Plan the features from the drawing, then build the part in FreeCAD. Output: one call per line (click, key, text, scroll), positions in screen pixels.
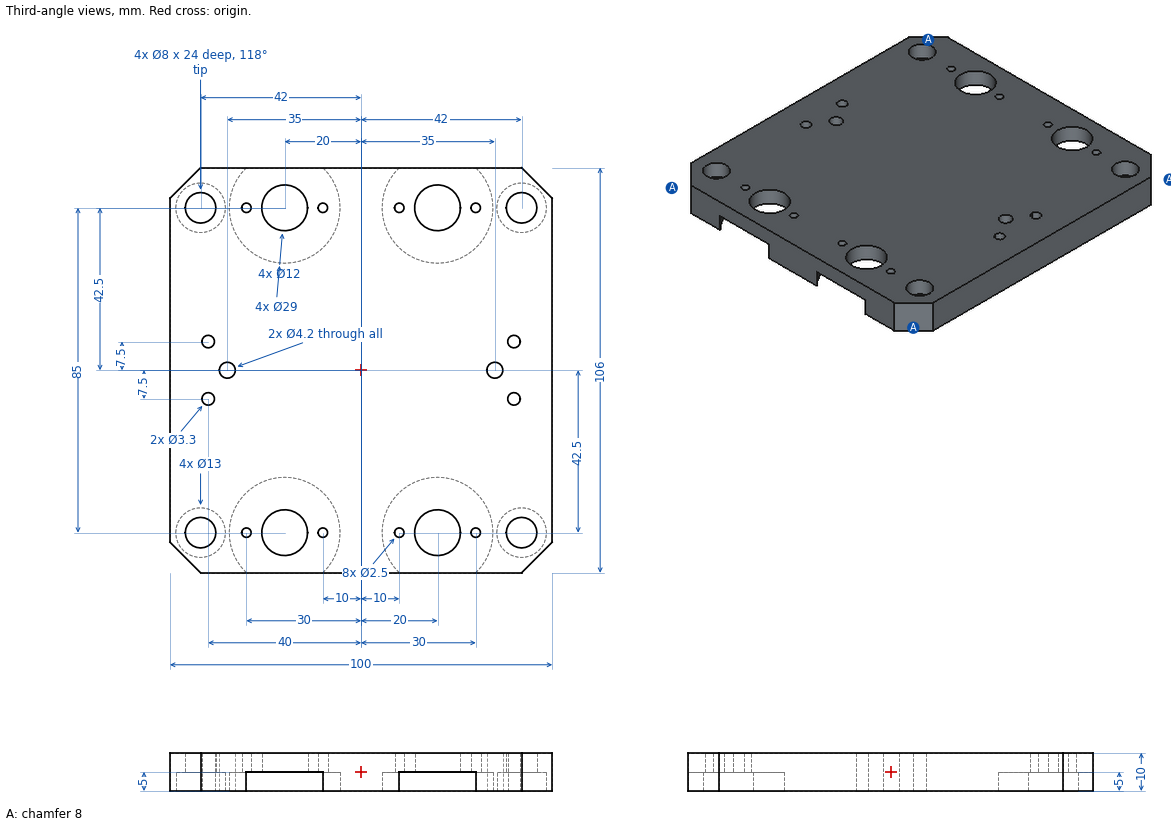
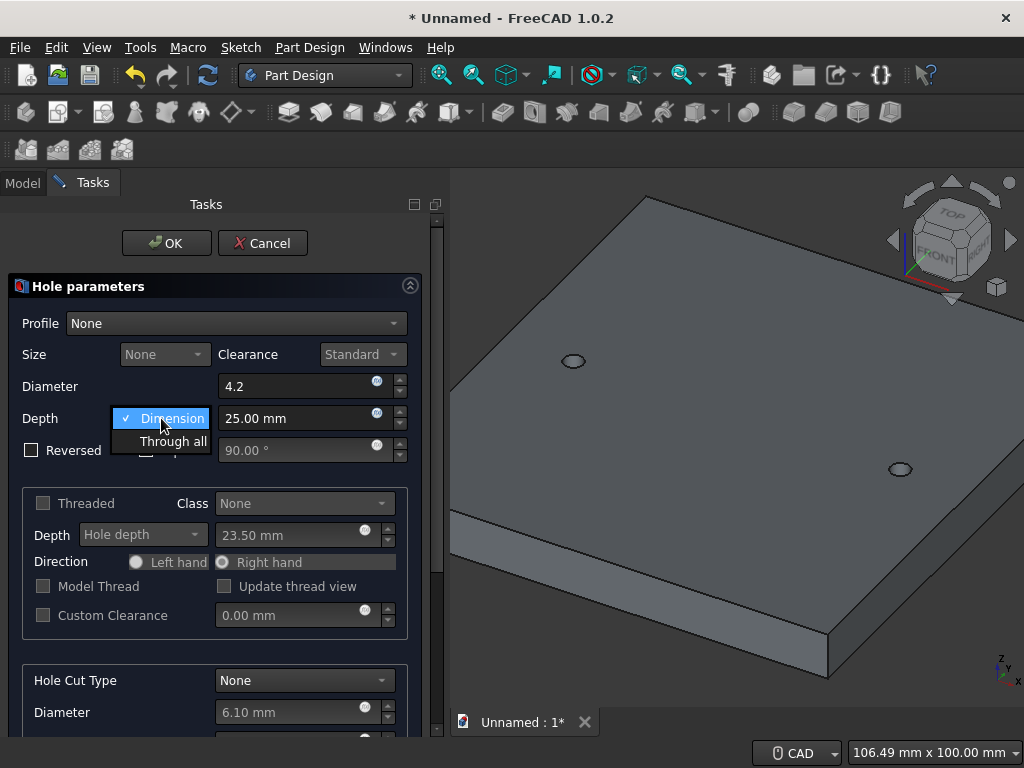
click(160, 442)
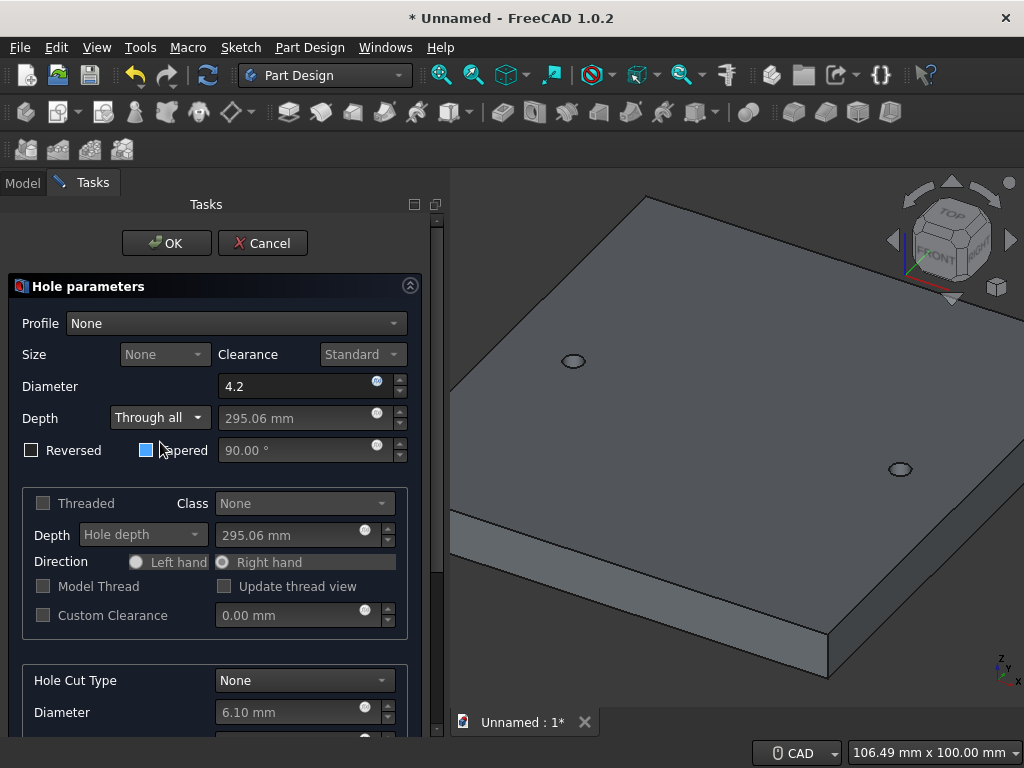
click(167, 243)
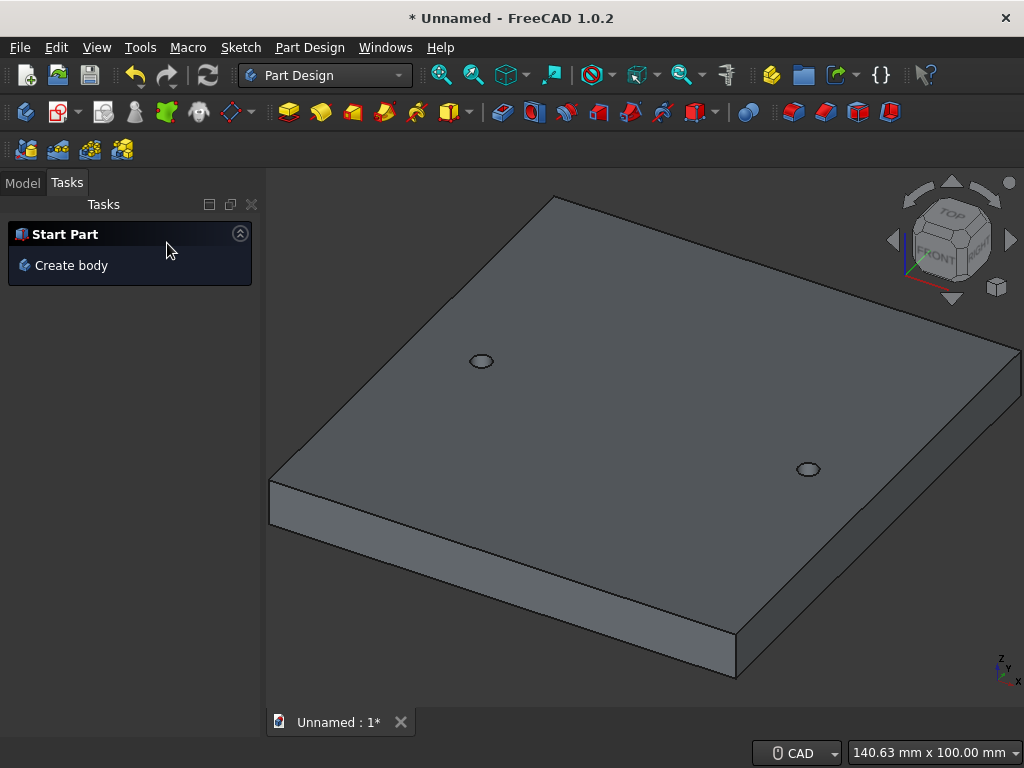
click(736, 656)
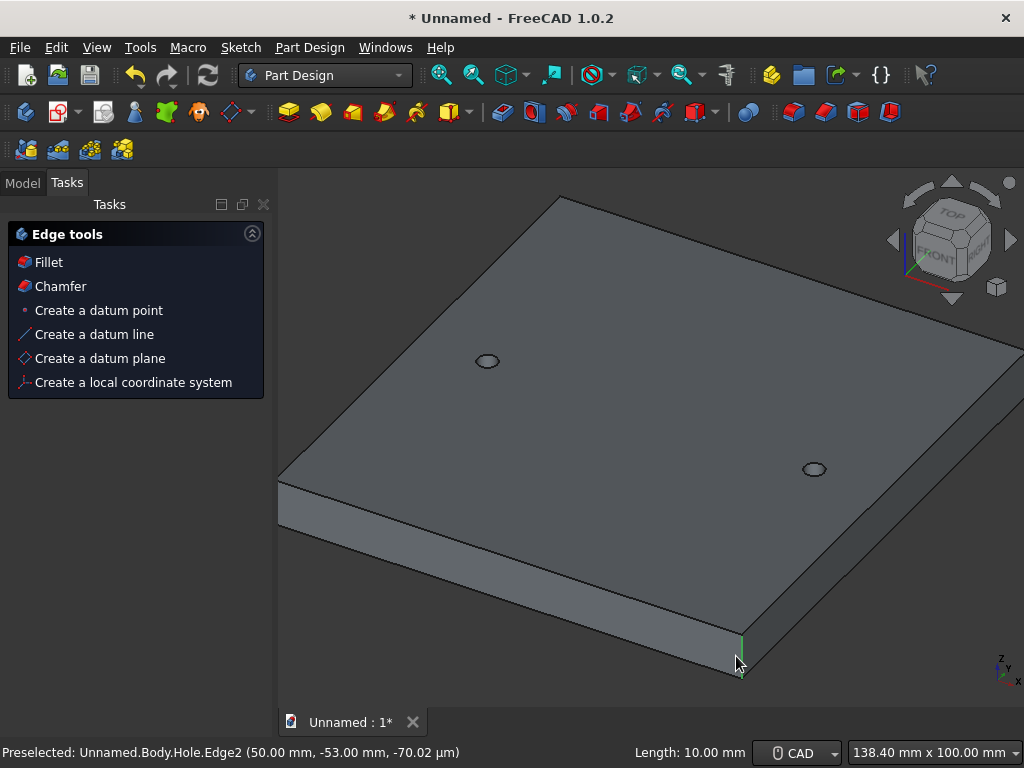
key(0)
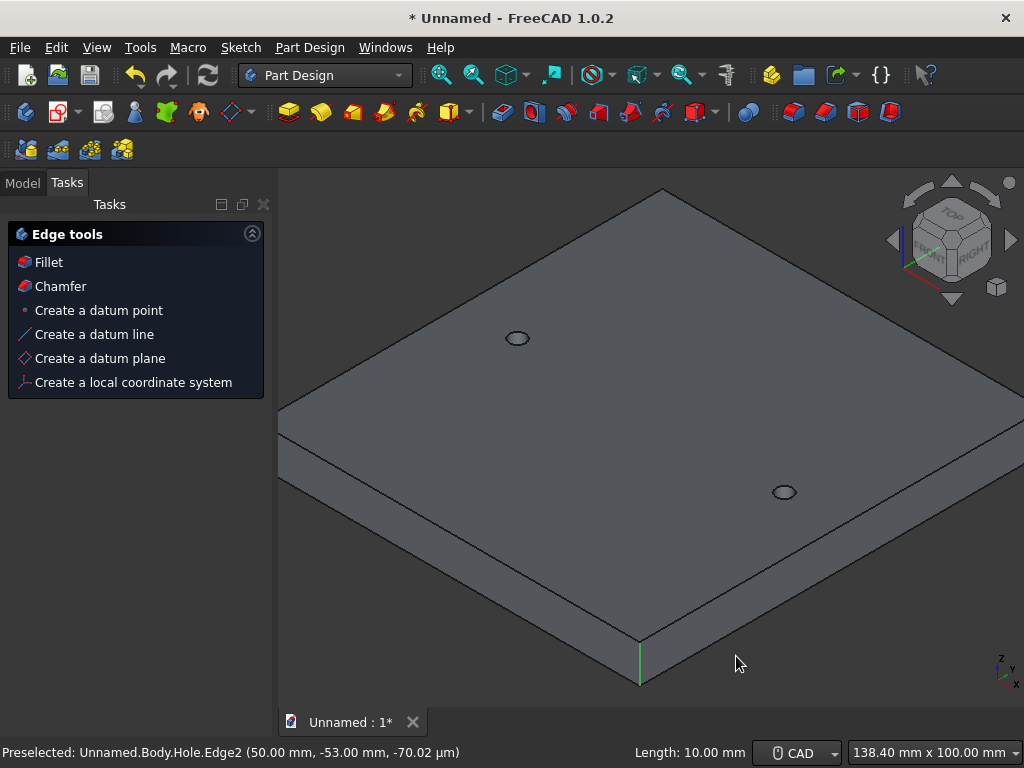
click(442, 76)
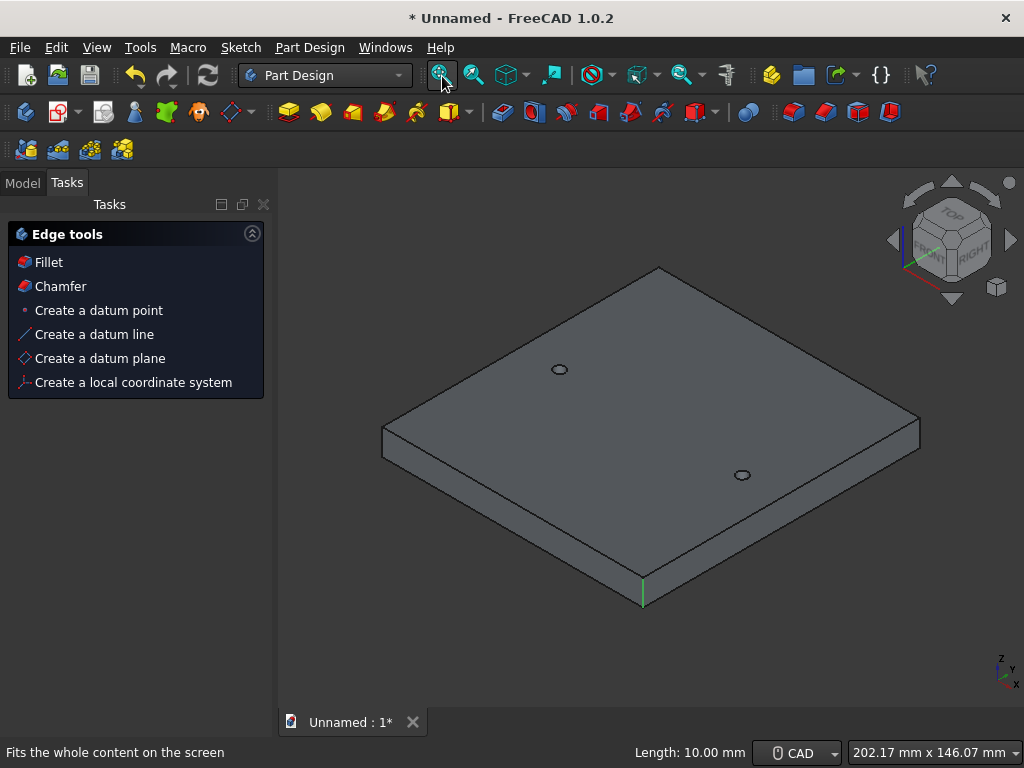
key(2)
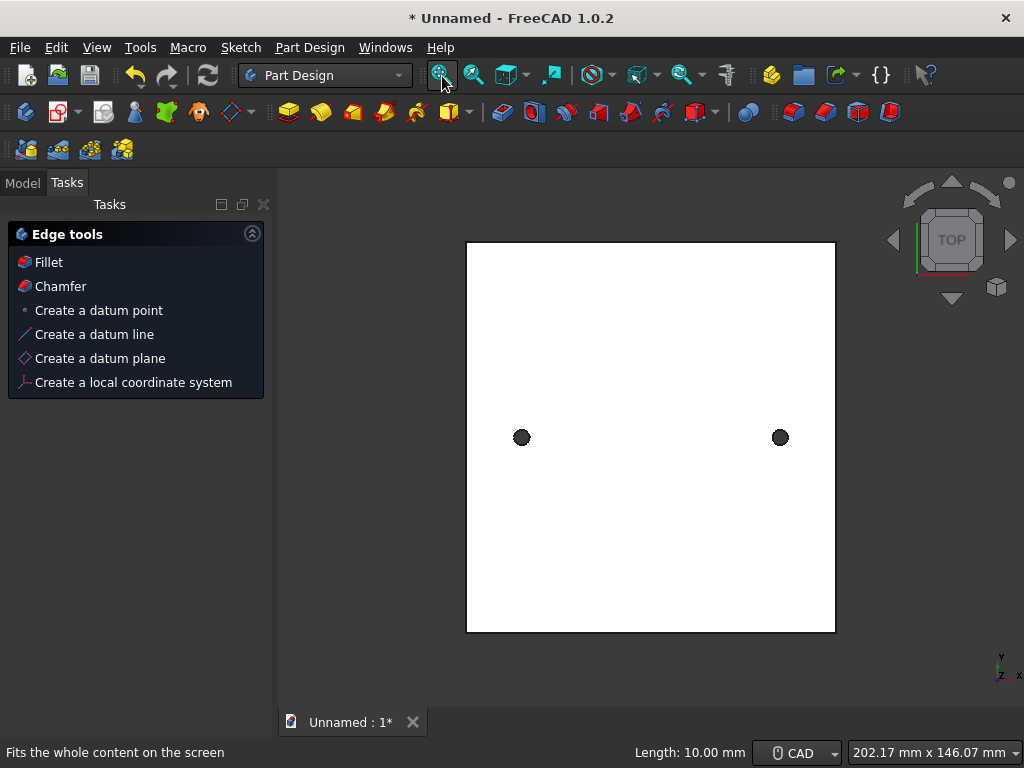
key(1)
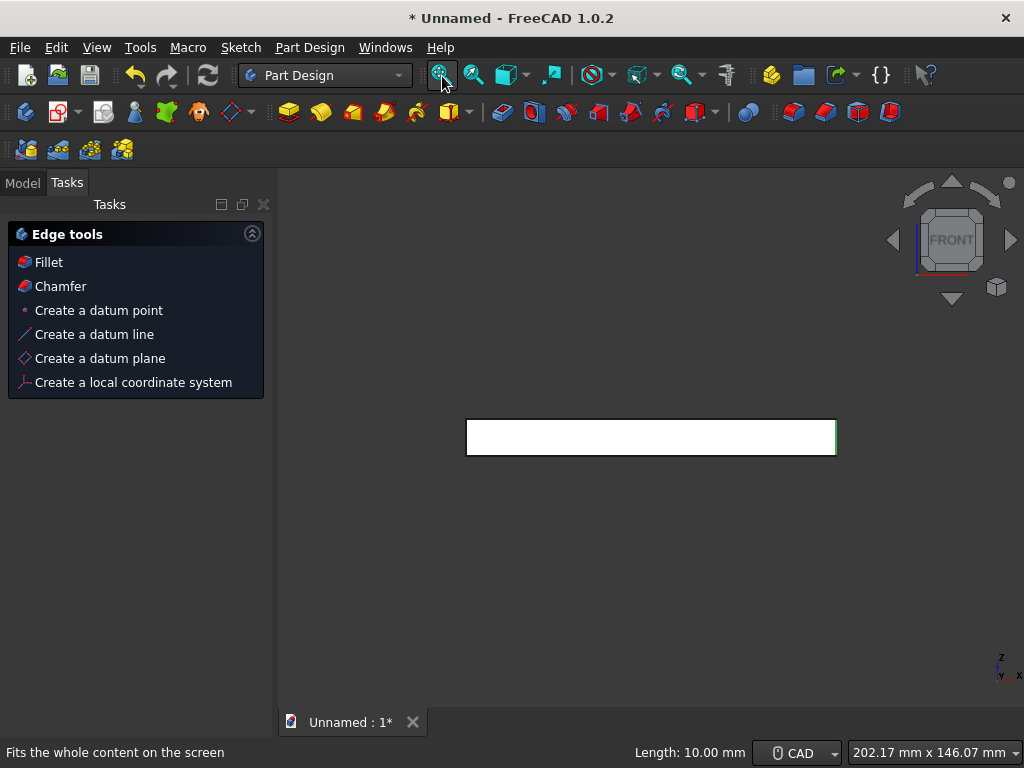
click(466, 436, ctrl)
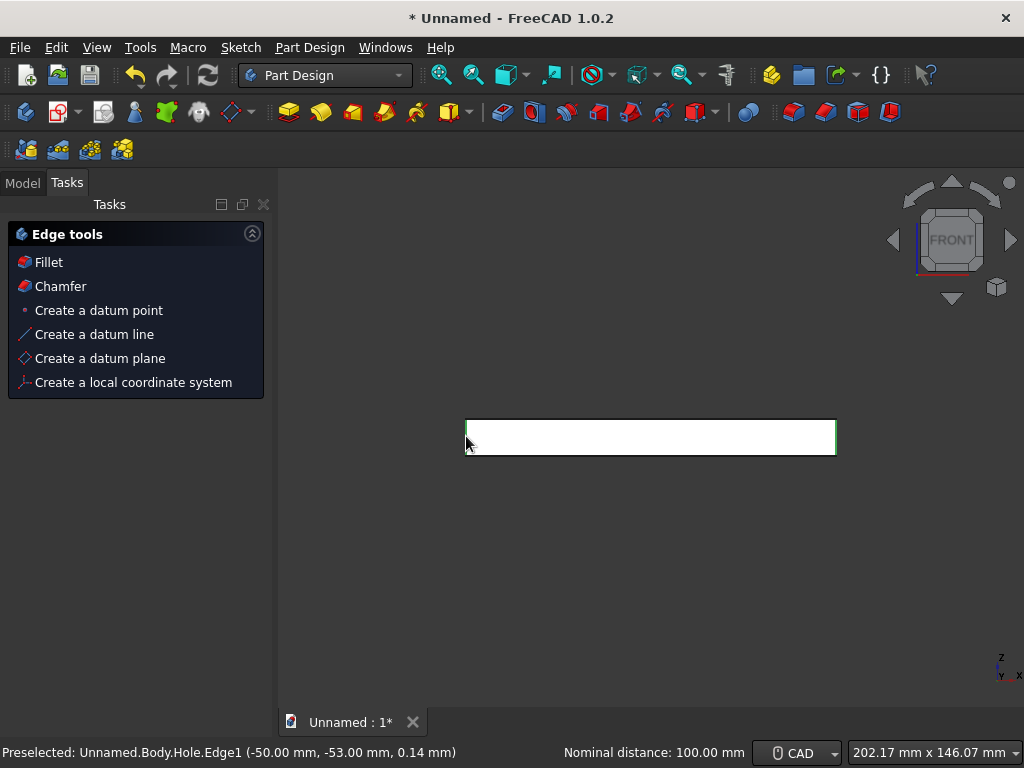
key(3)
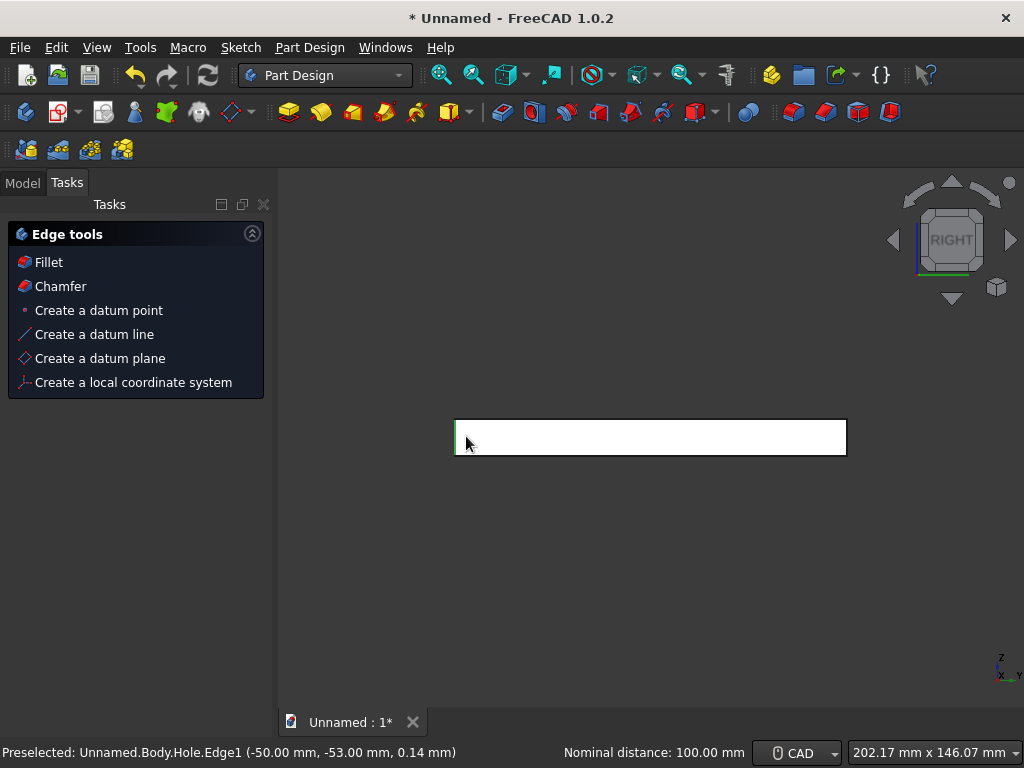
click(847, 436, ctrl)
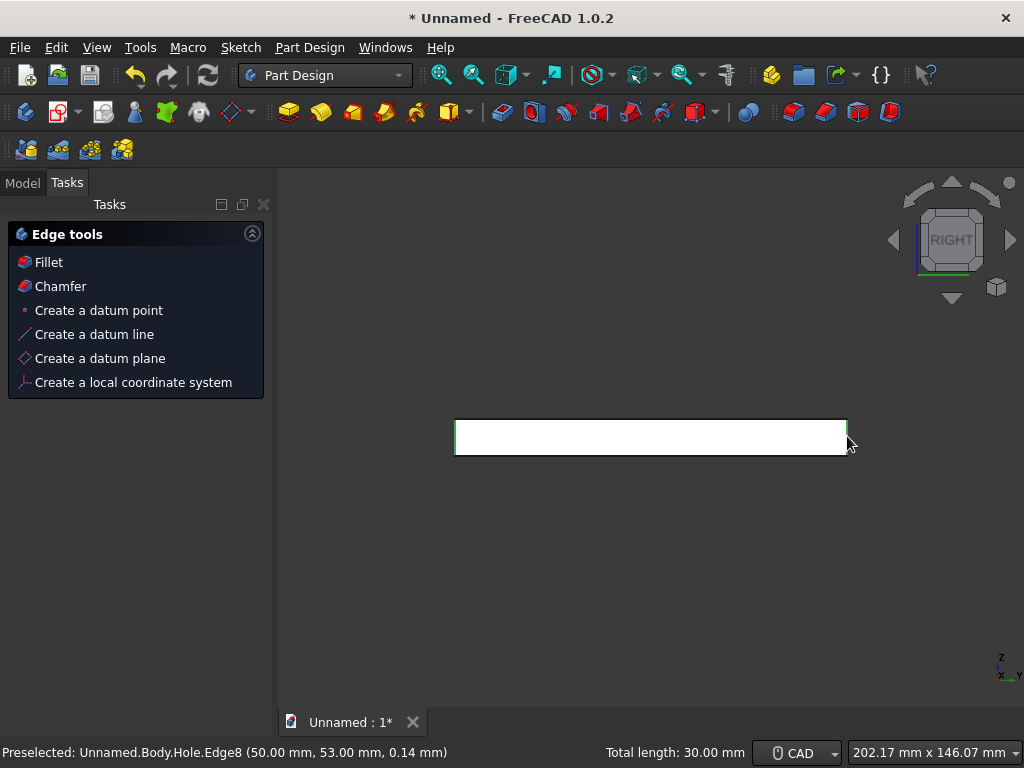
key(5)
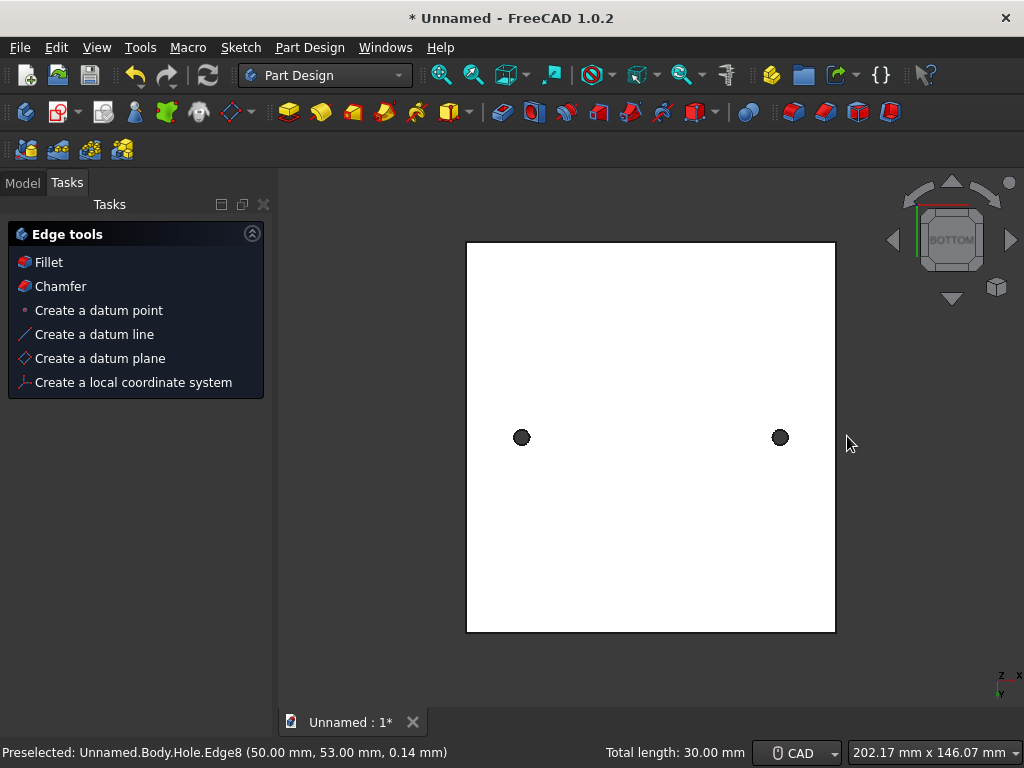
key(4)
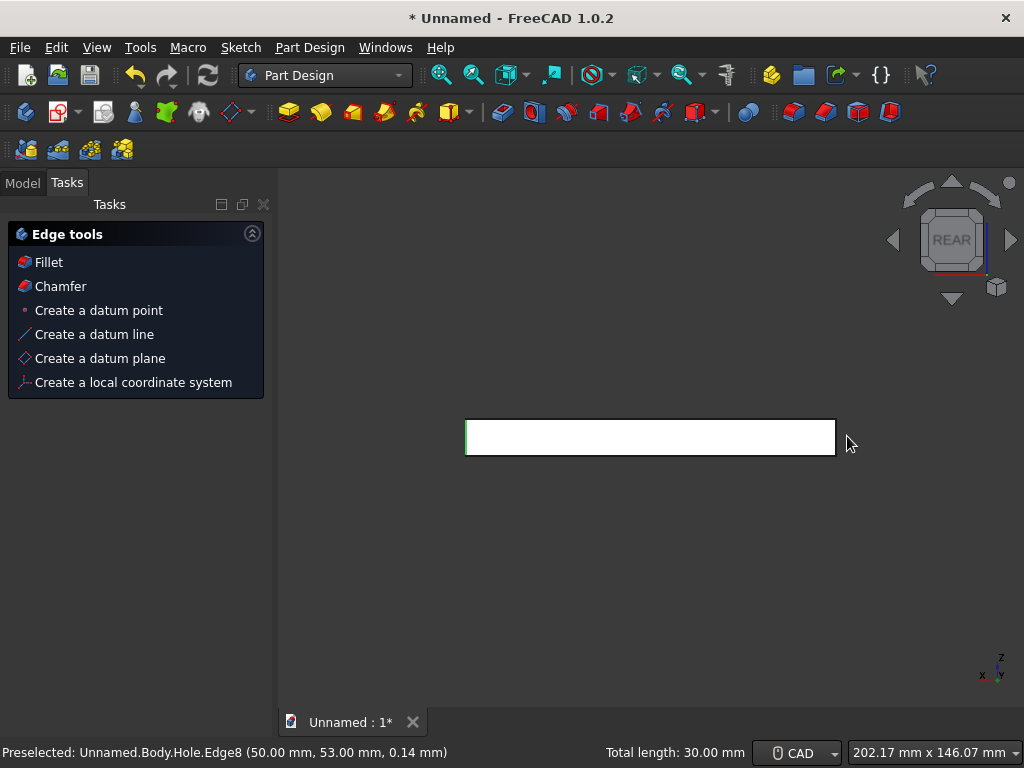
click(836, 436, ctrl)